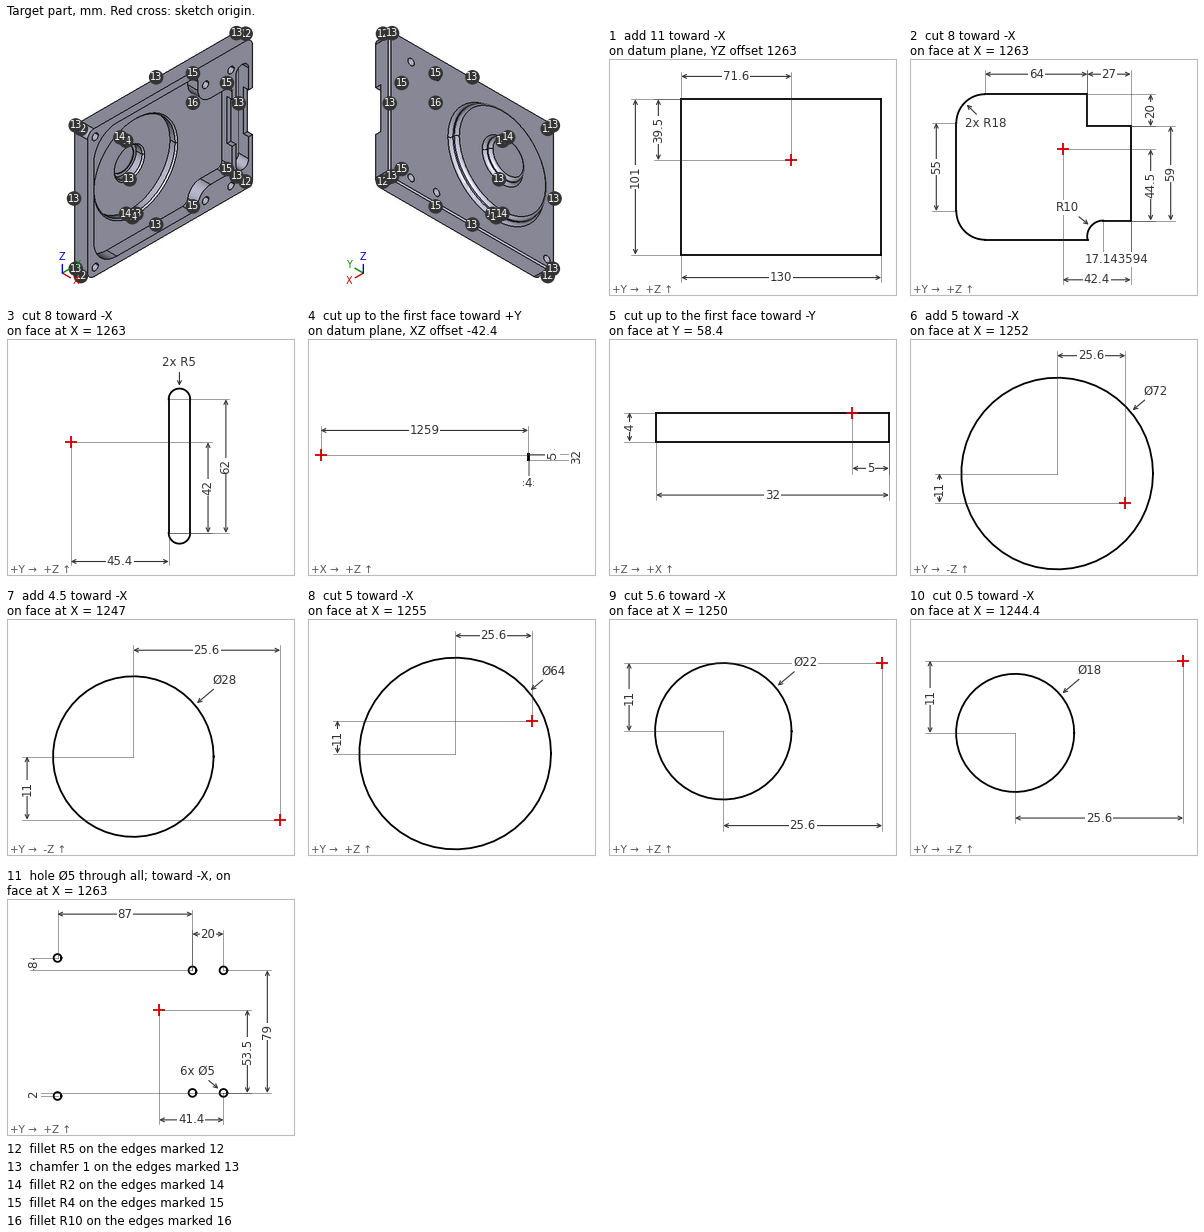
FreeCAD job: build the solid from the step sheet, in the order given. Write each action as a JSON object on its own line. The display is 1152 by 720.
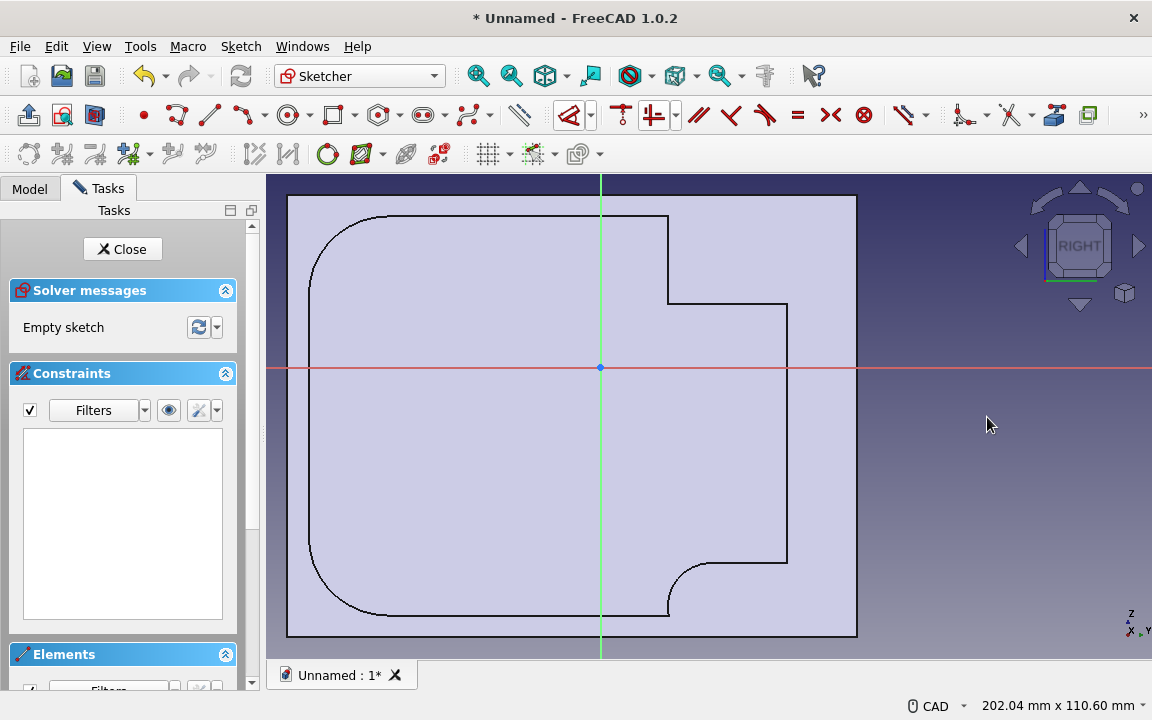
{"action": "left_click", "coordinate": [422, 116]}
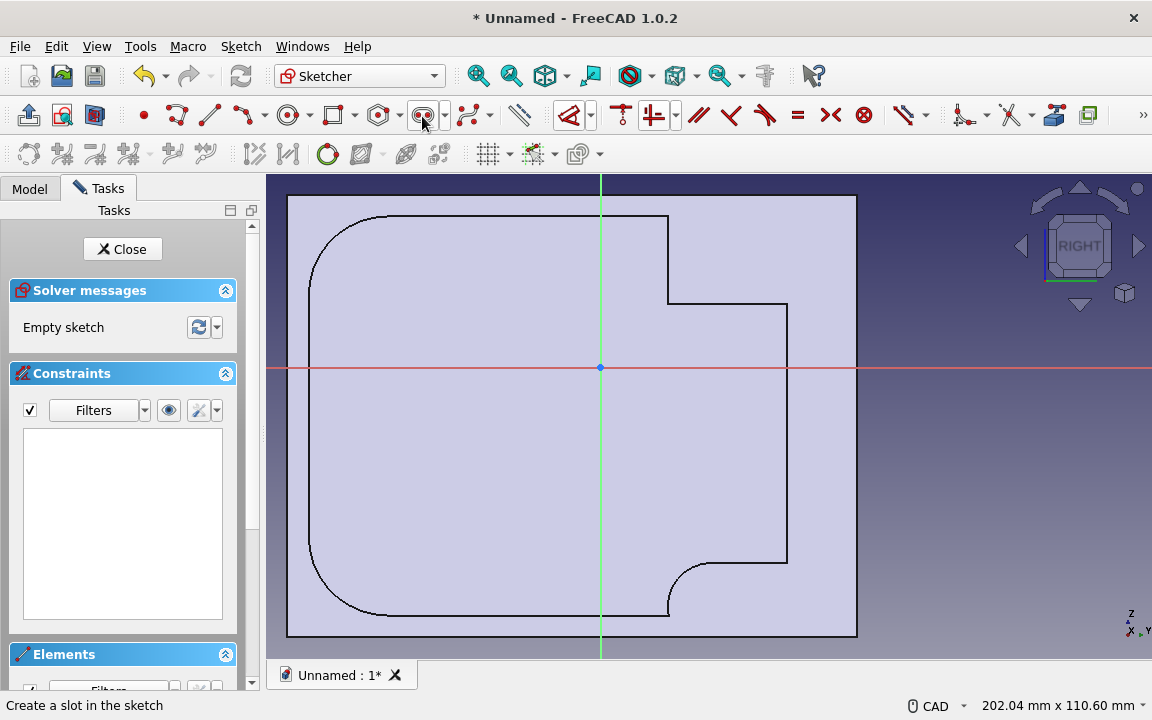
{"action": "left_click", "coordinate": [822, 552]}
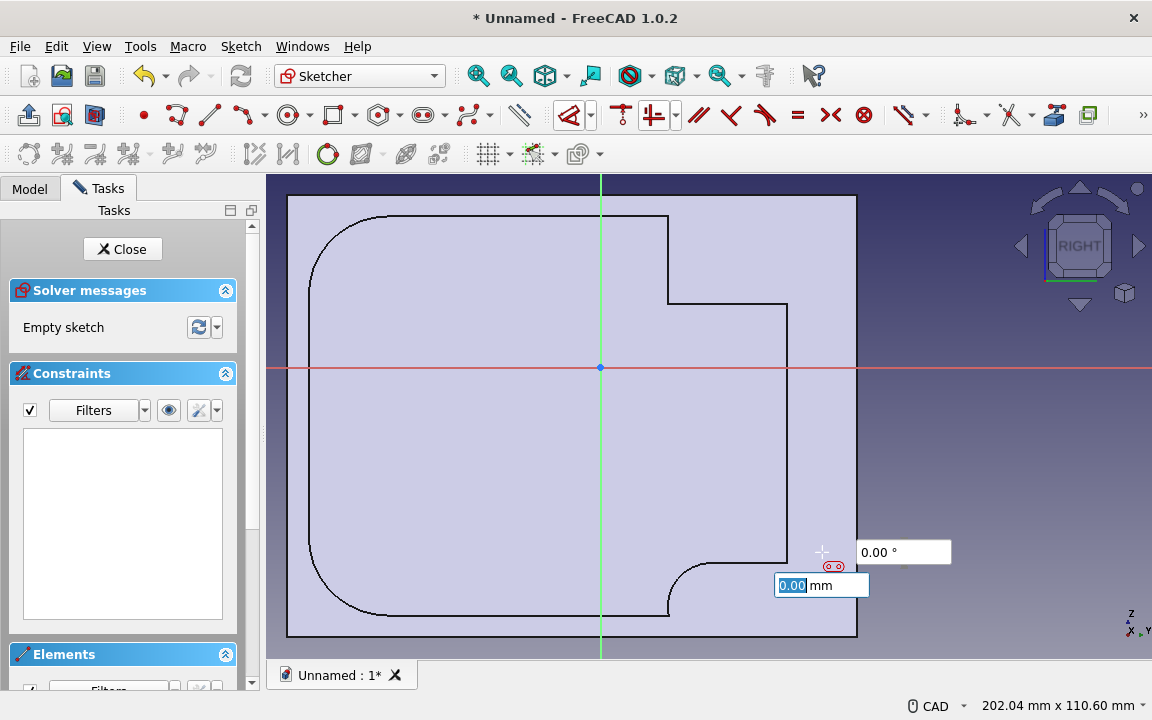
{"action": "left_click", "coordinate": [822, 280]}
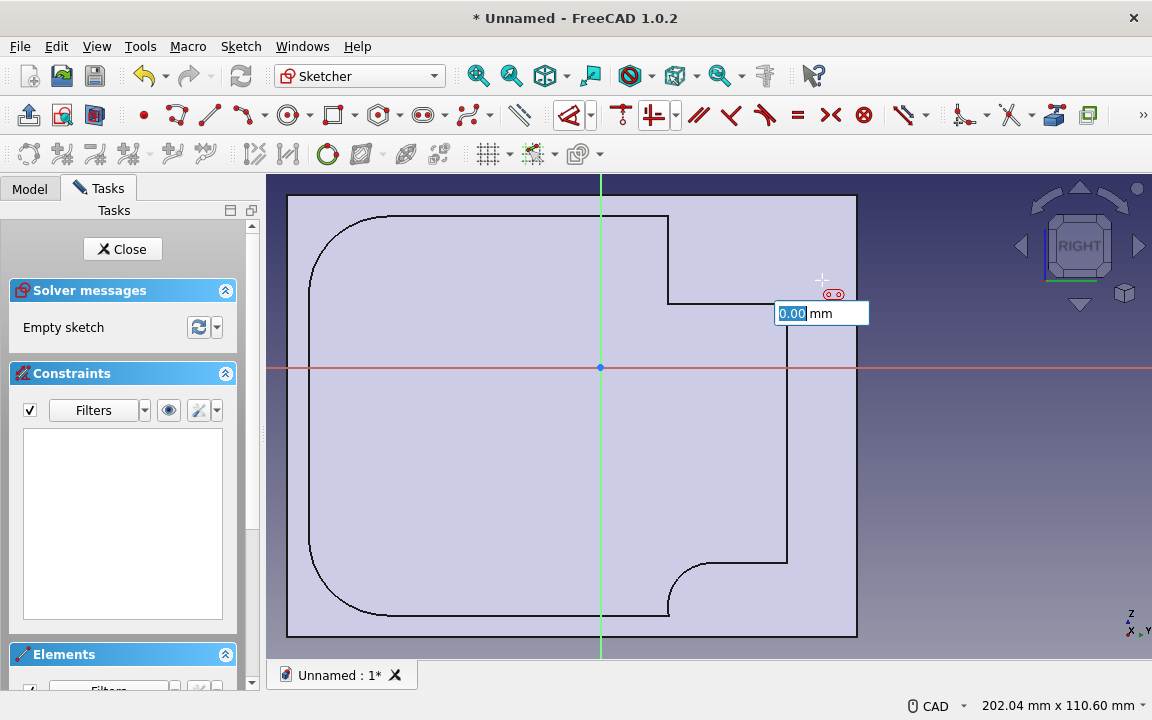
{"action": "left_click", "coordinate": [844, 416]}
{"action": "key", "text": "Escape"}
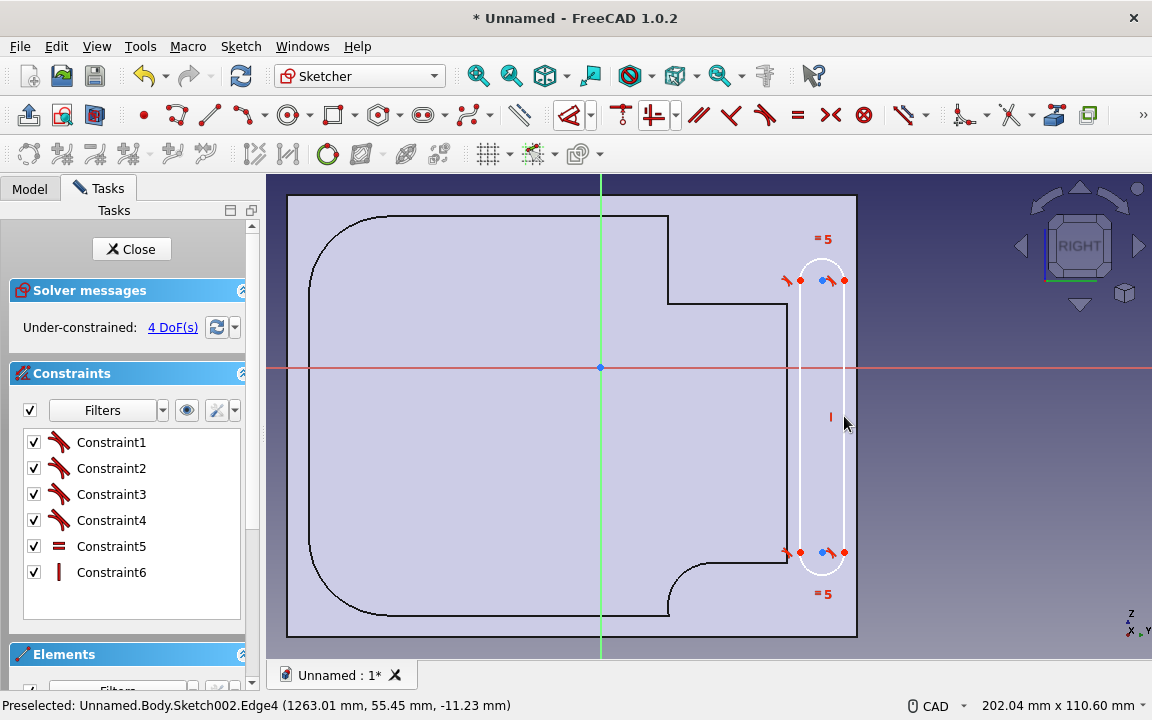
{"action": "scroll", "coordinate": [809, 571], "scroll_direction": "up", "scroll_amount": 3}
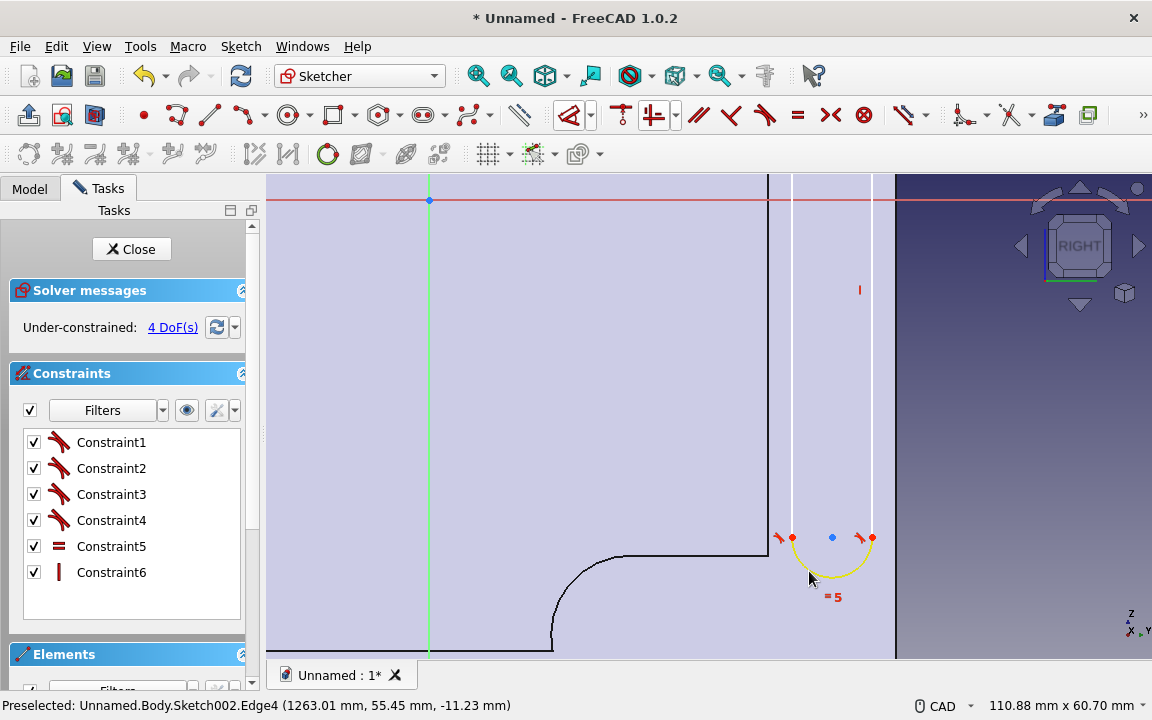
{"action": "left_click", "coordinate": [809, 570]}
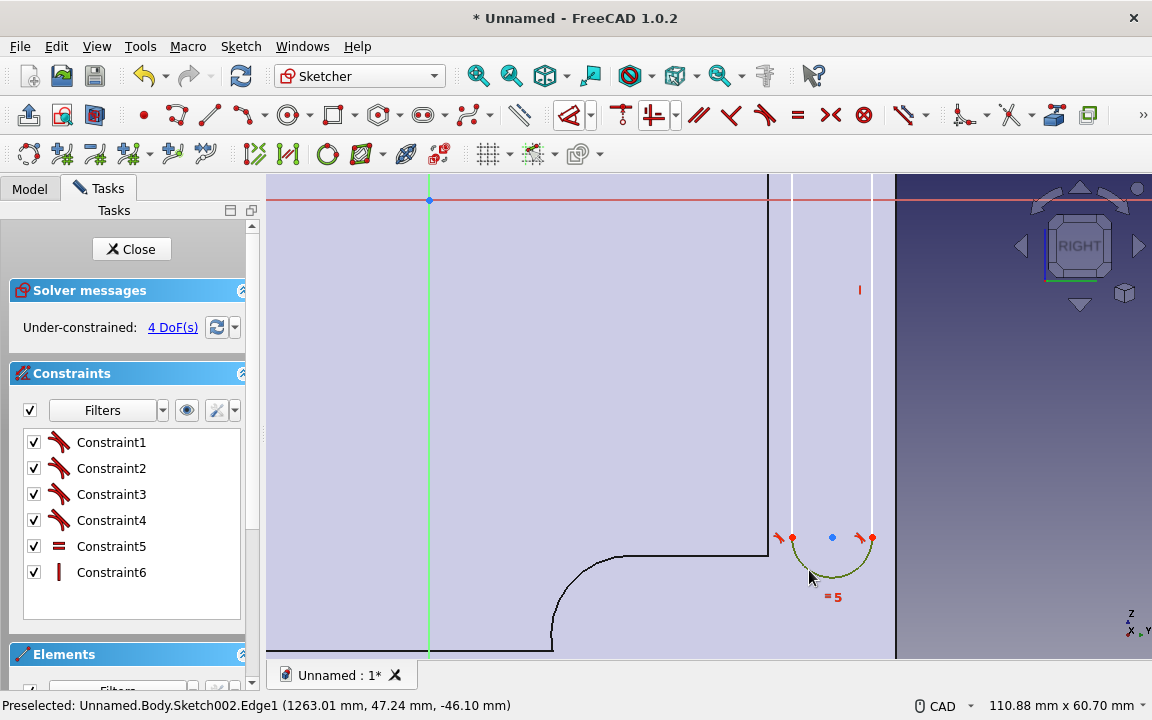
{"action": "key", "text": "k r"}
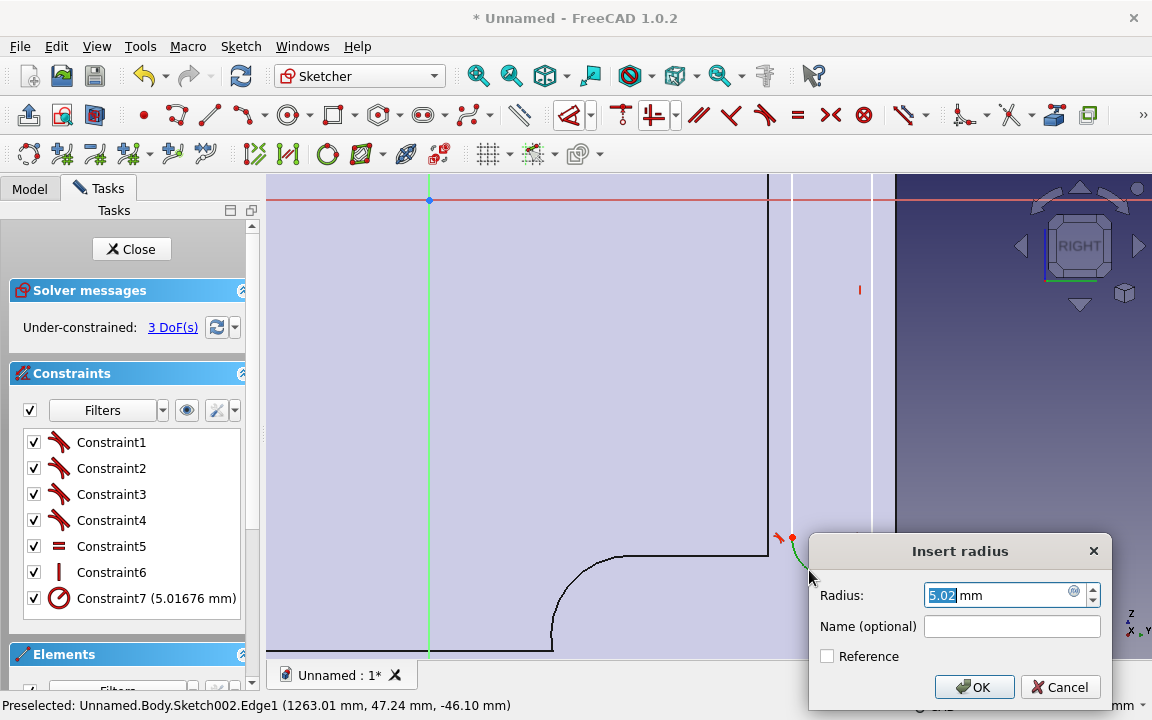
{"action": "type", "text": "5"}
{"action": "key", "text": "Return"}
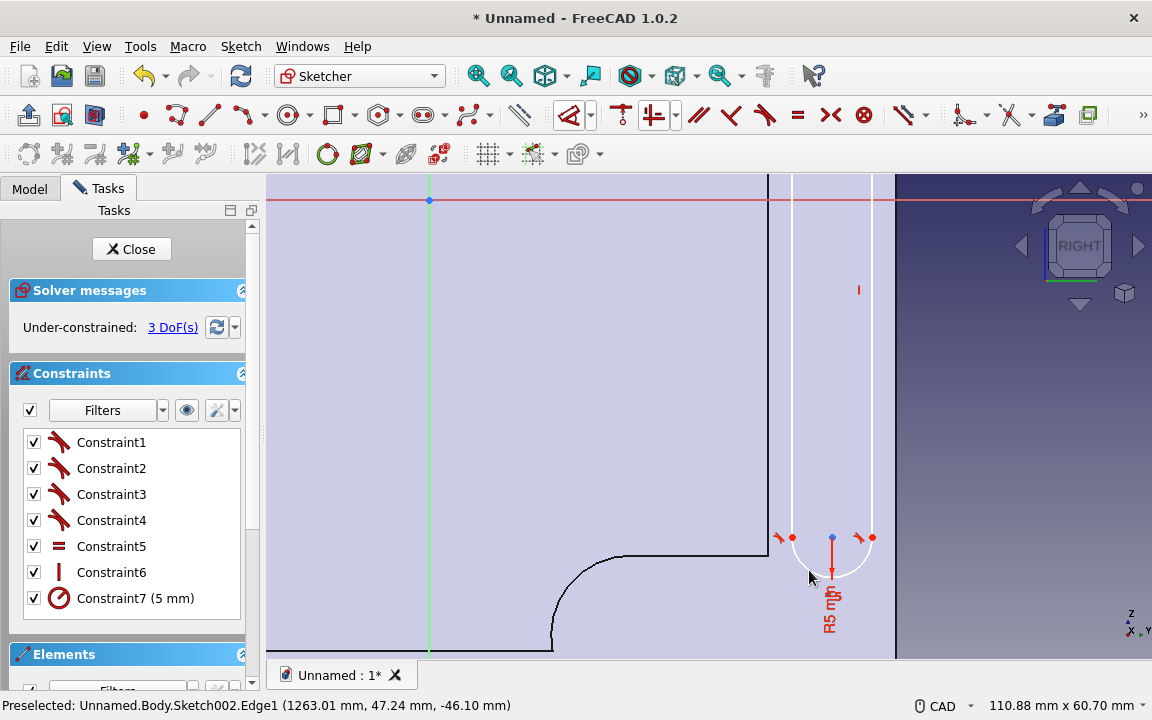
{"action": "left_click", "coordinate": [792, 389]}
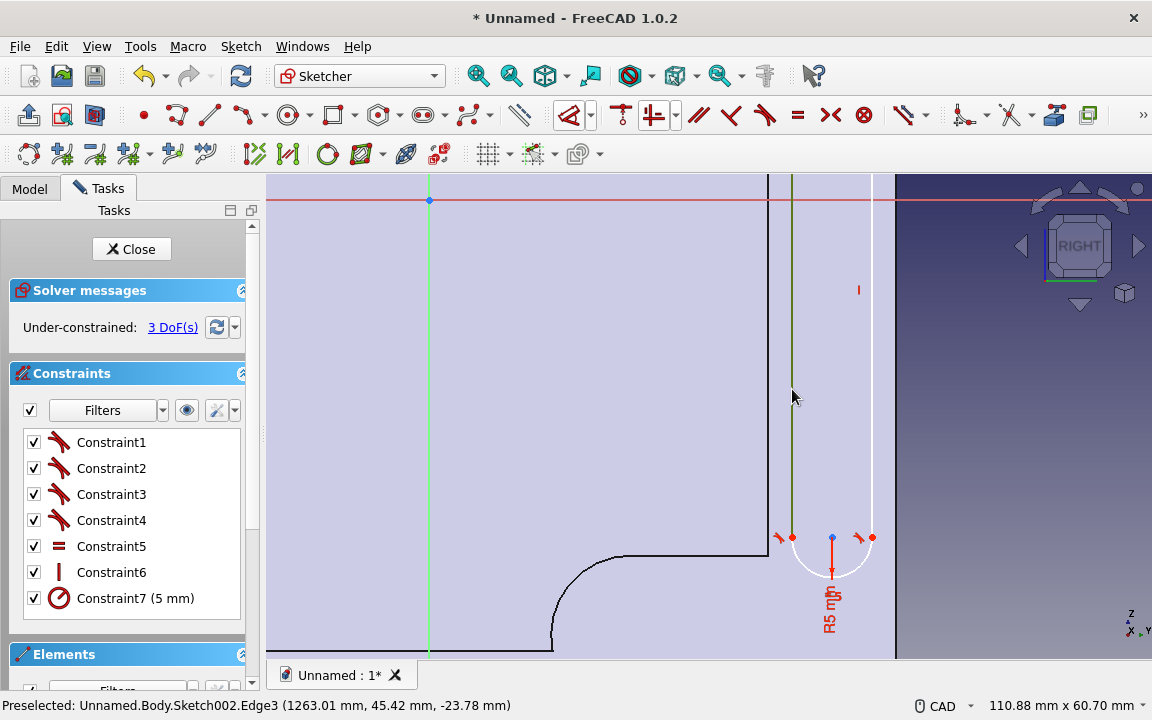
{"action": "key", "text": "i"}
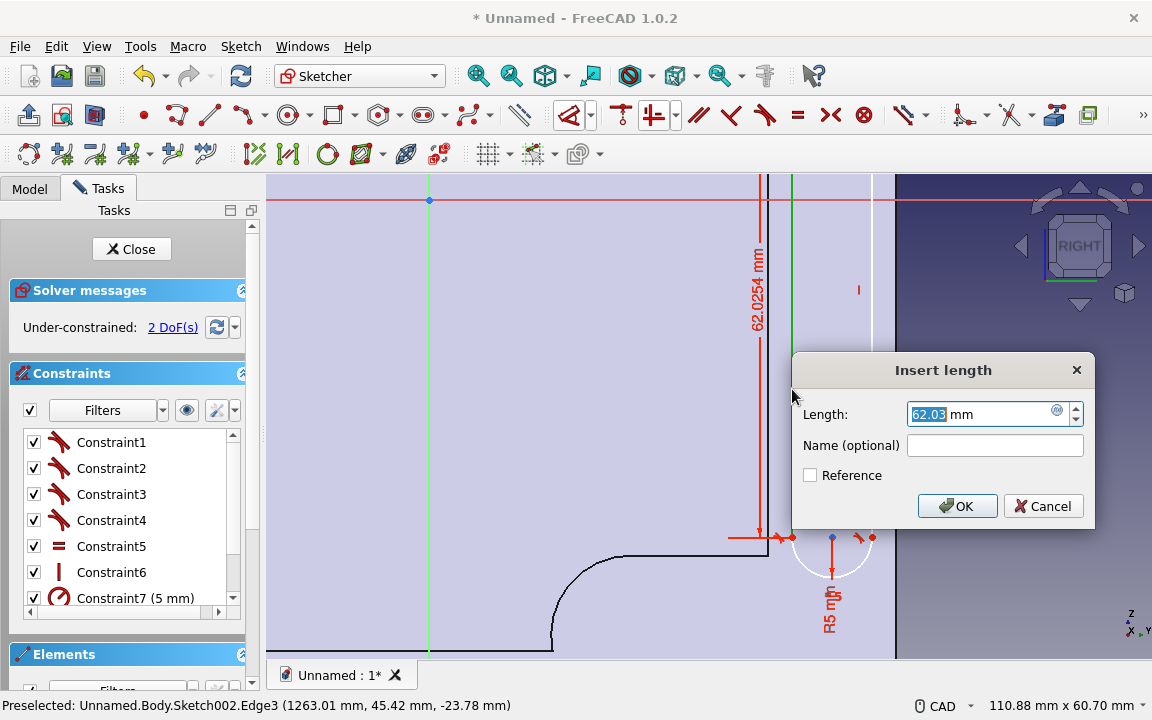
{"action": "type", "text": "62"}
{"action": "key", "text": "Return"}